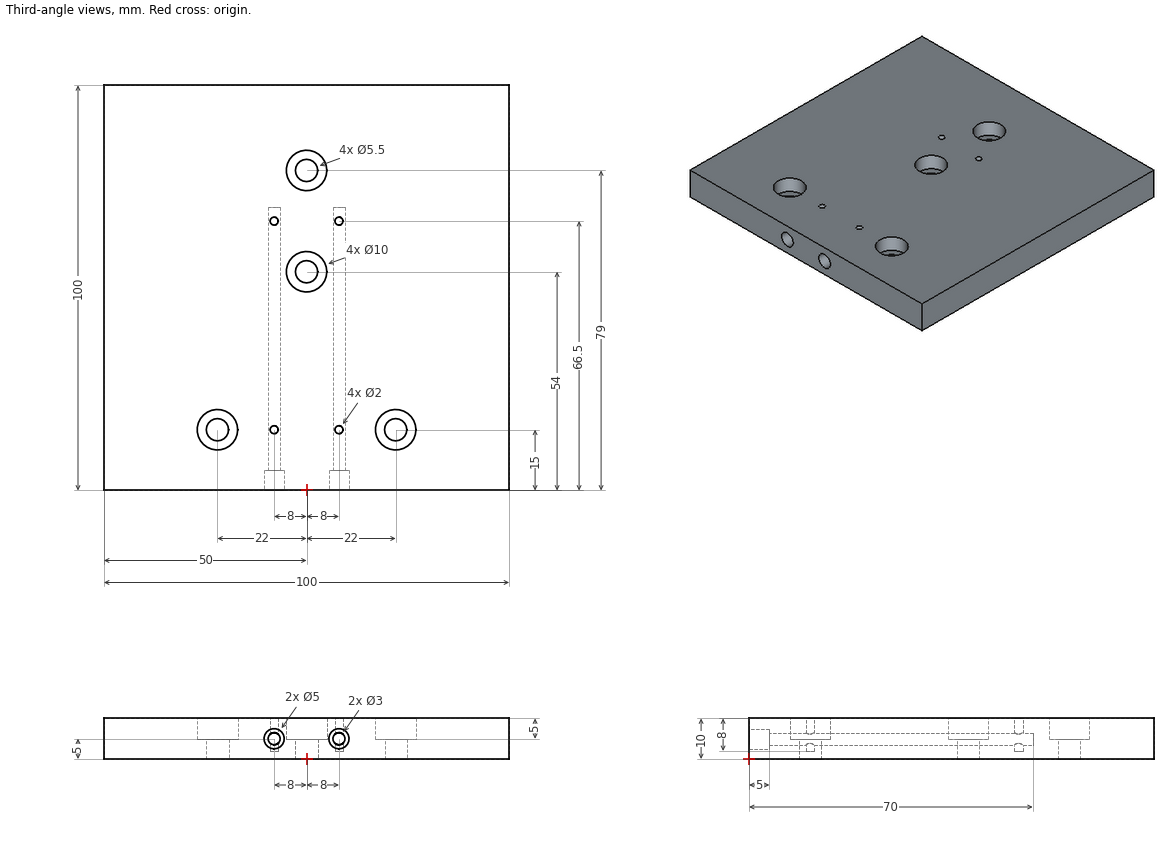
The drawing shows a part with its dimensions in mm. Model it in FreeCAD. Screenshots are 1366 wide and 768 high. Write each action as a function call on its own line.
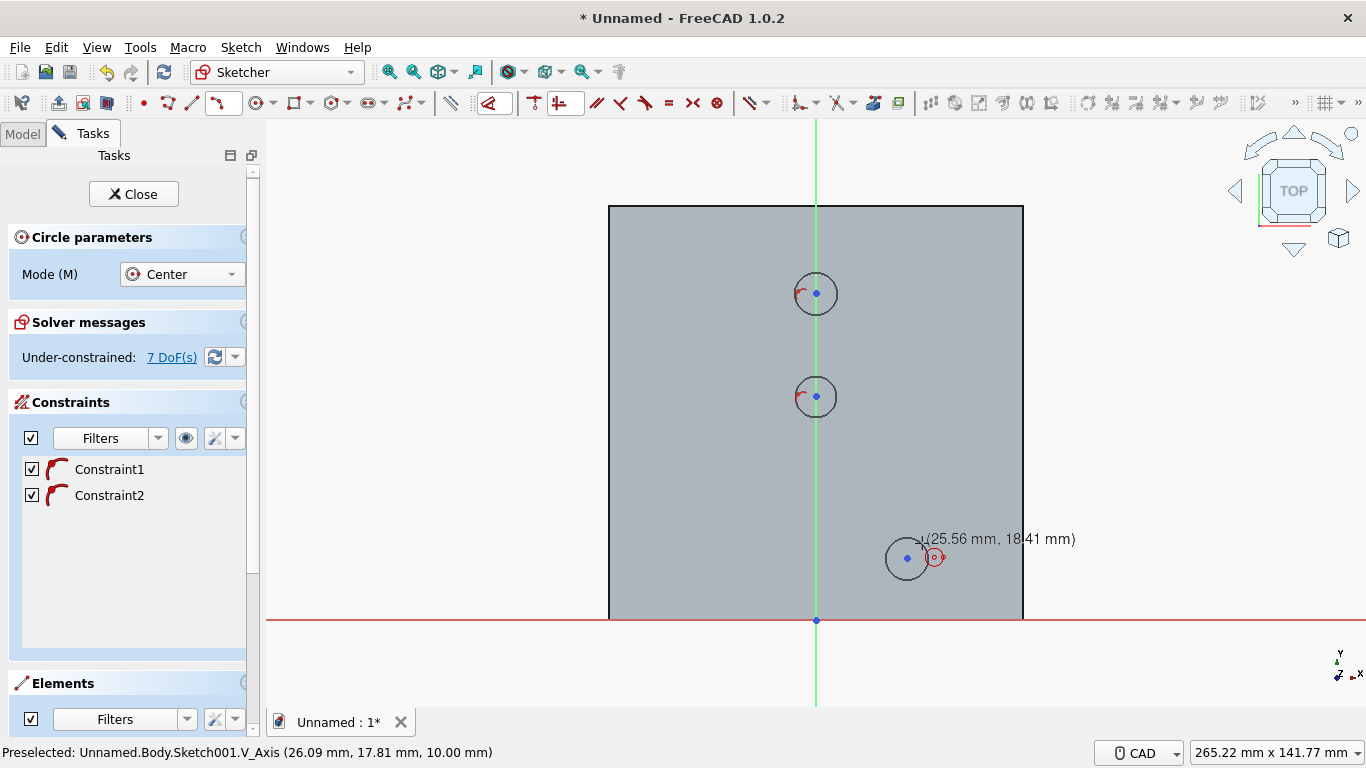
click(725, 558)
click(739, 543)
key(Escape)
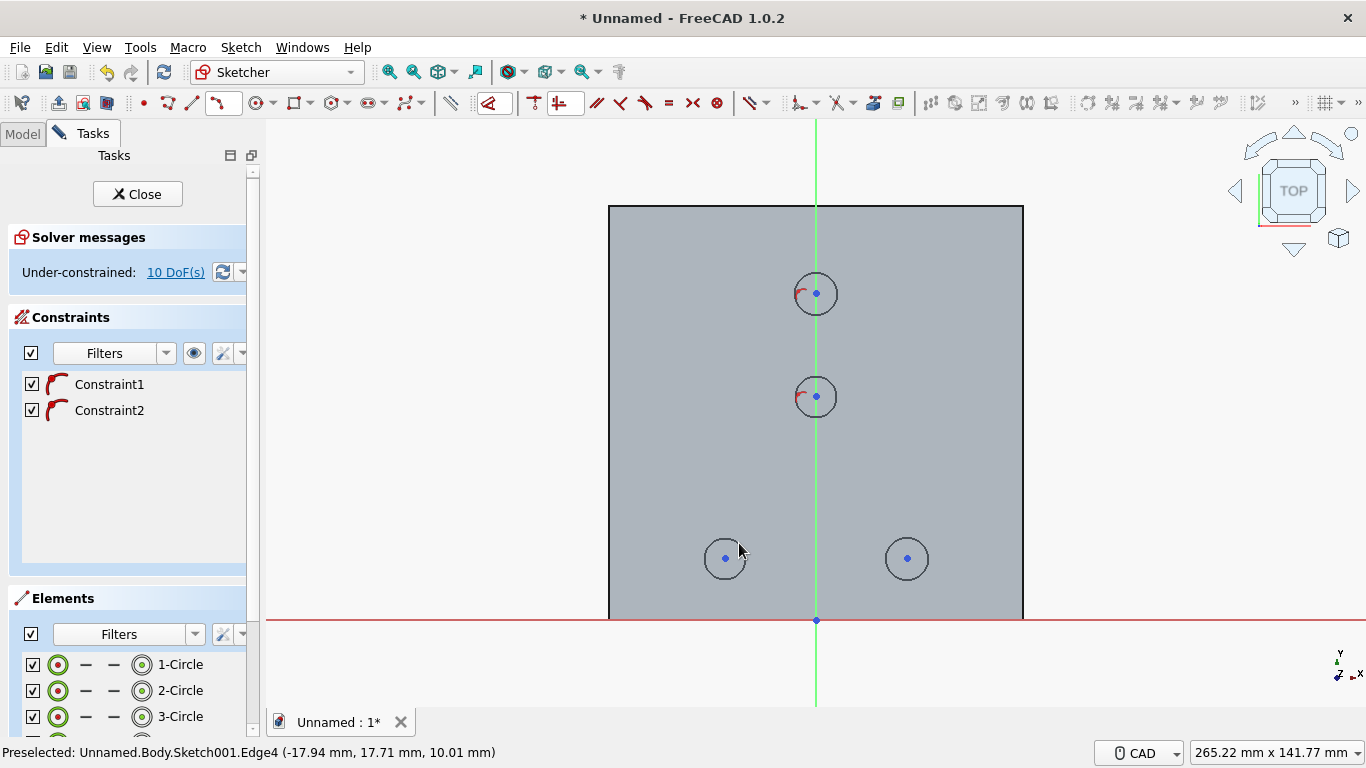
click(830, 382)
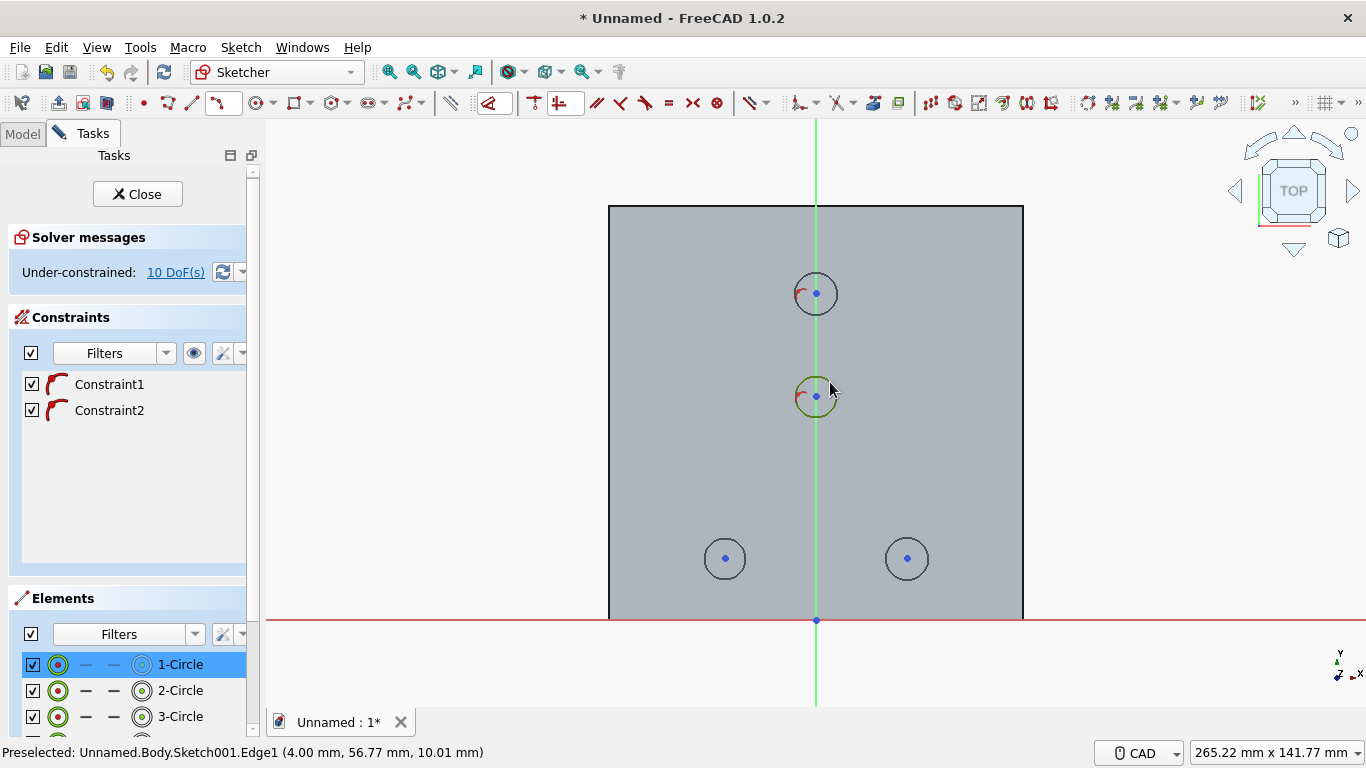
click(831, 279)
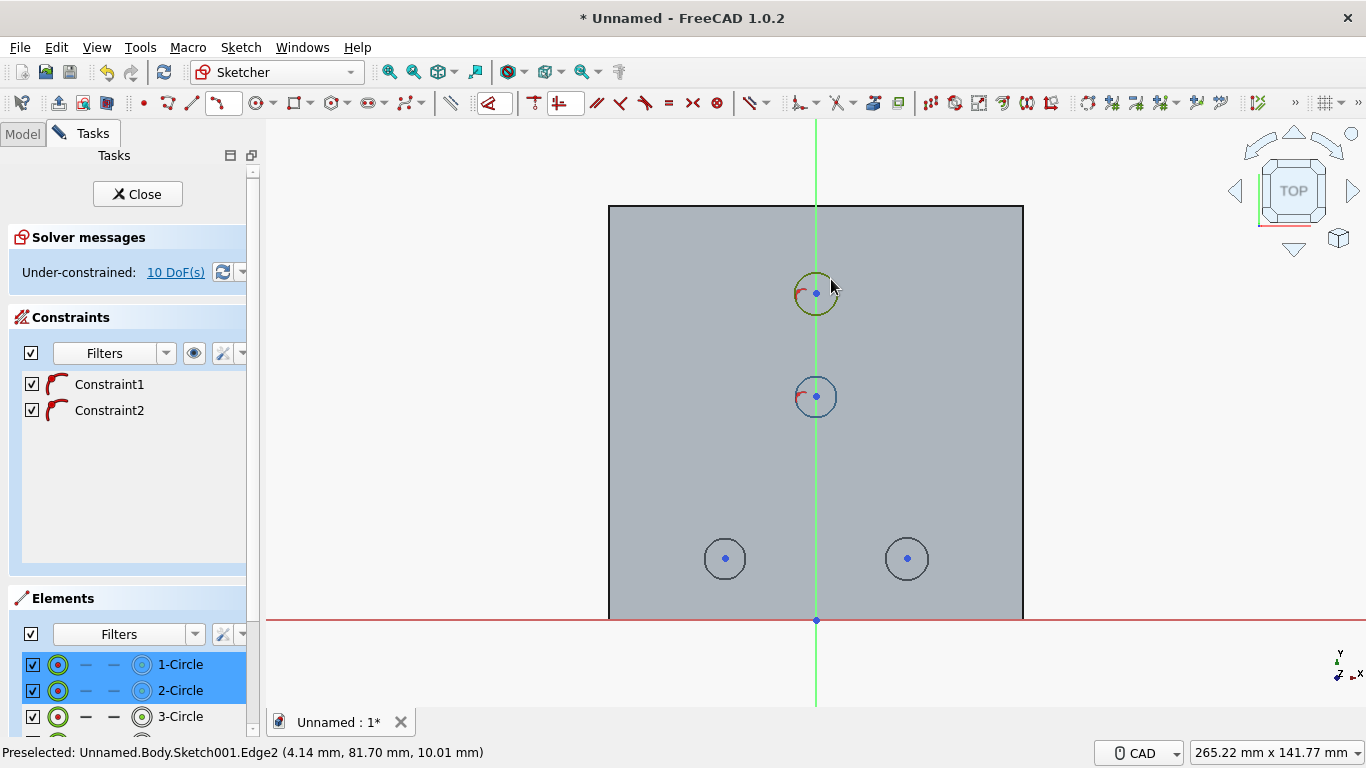
click(922, 544)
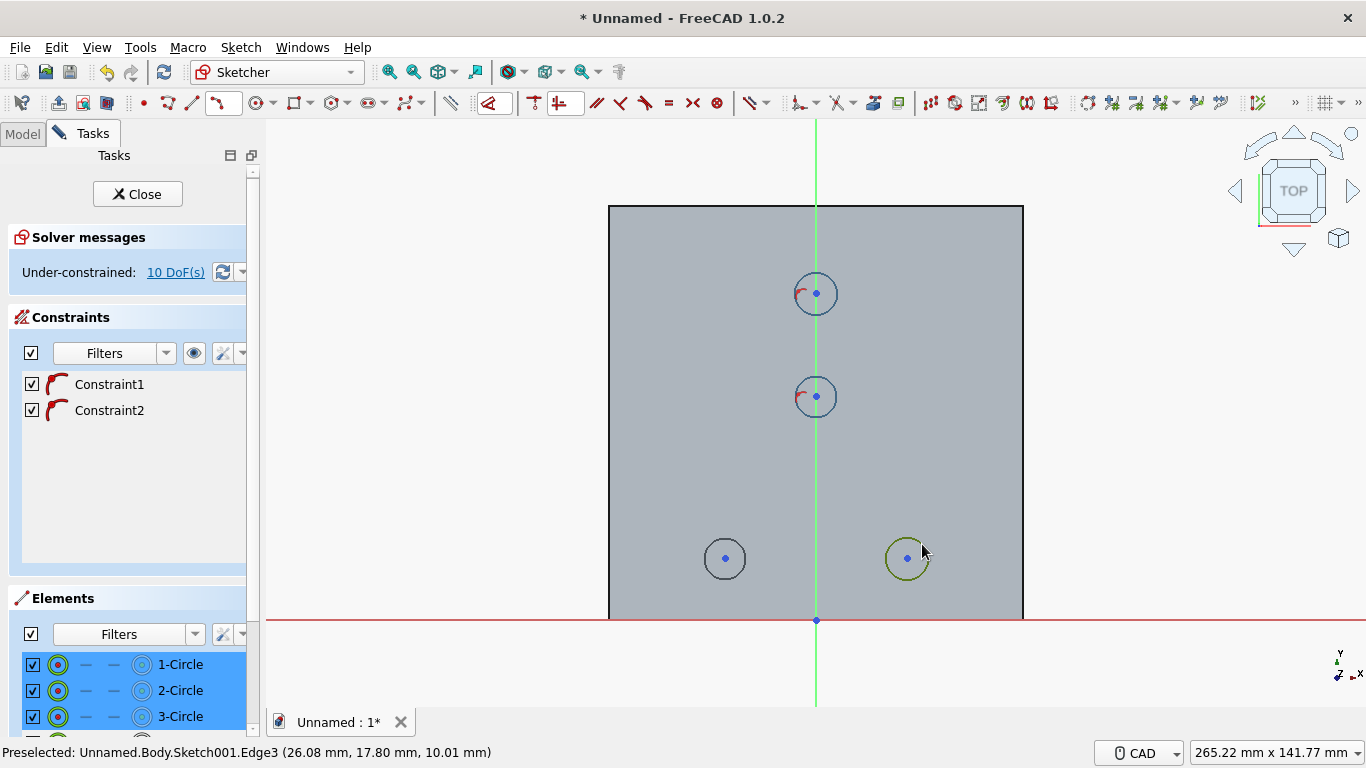
click(739, 544)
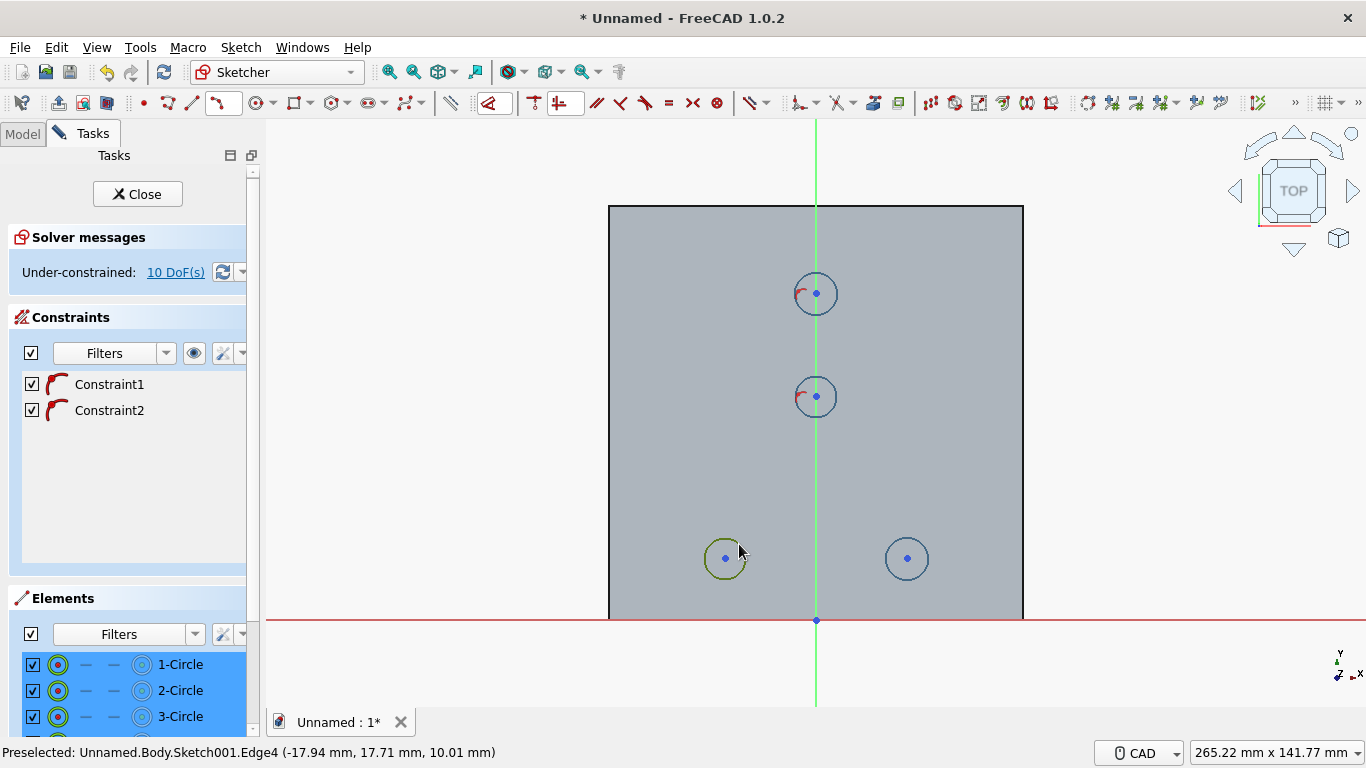
click(670, 104)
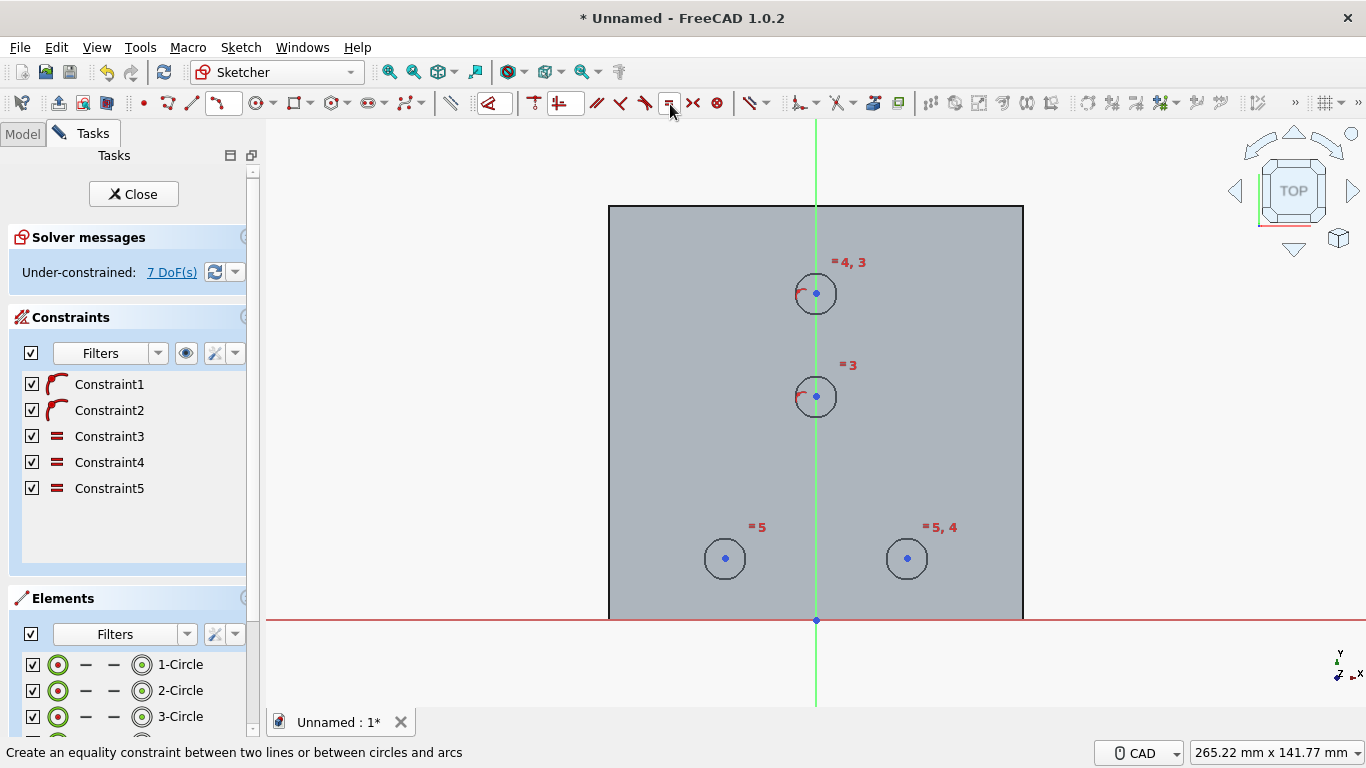
click(830, 382)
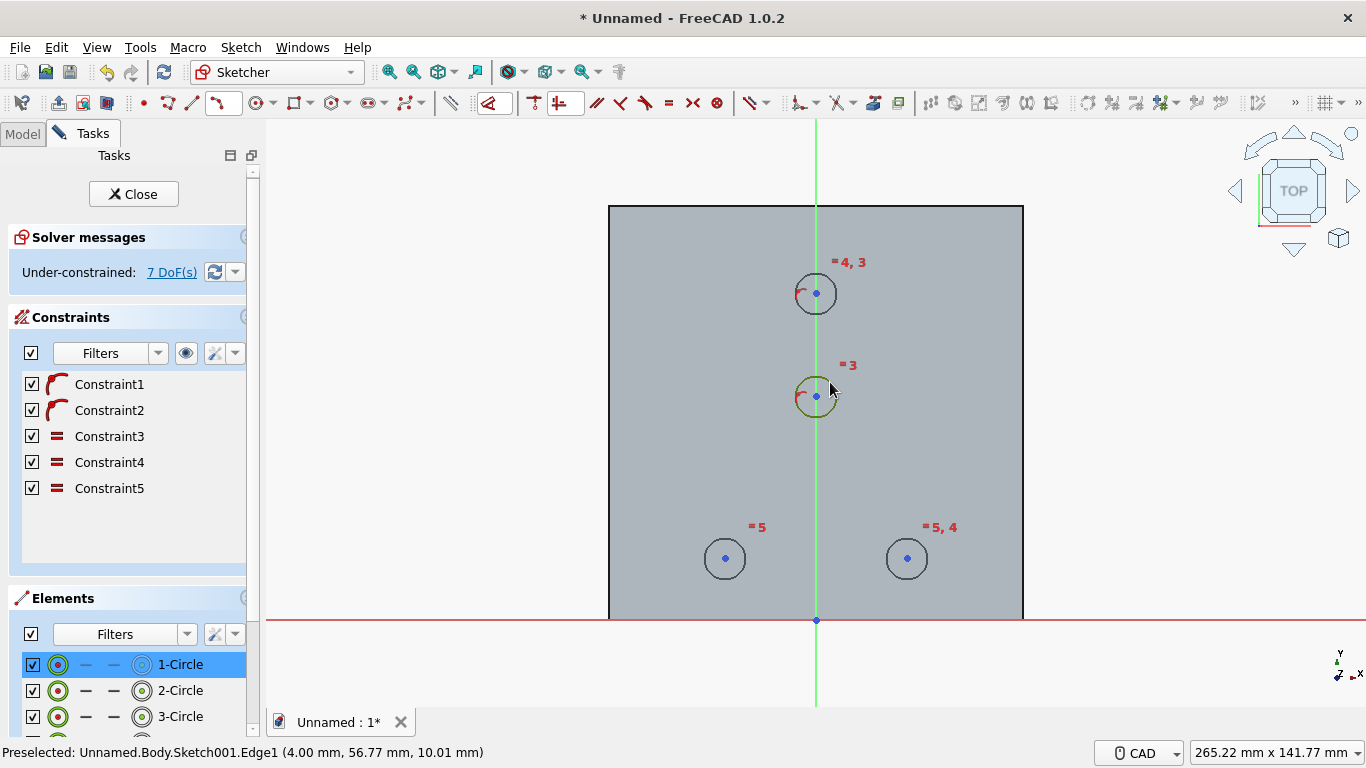
click(506, 104)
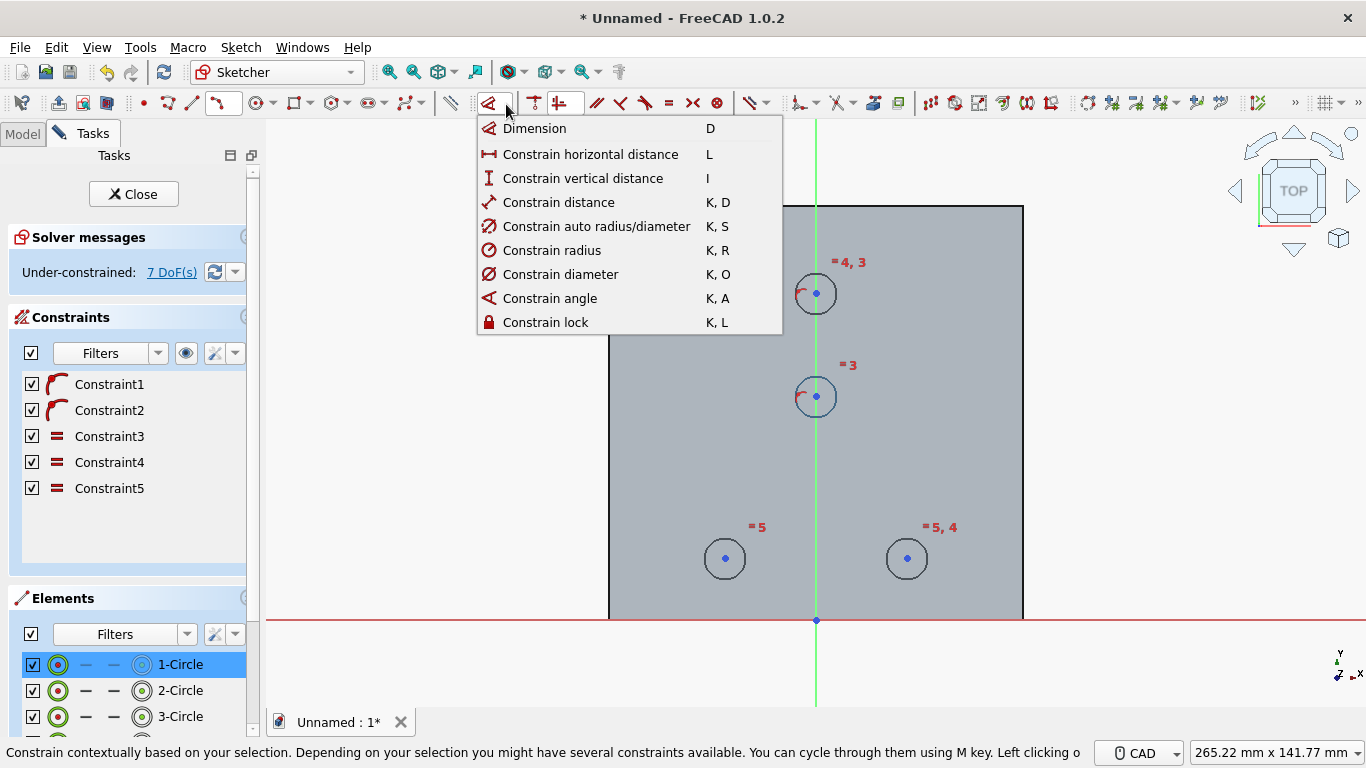
click(630, 274)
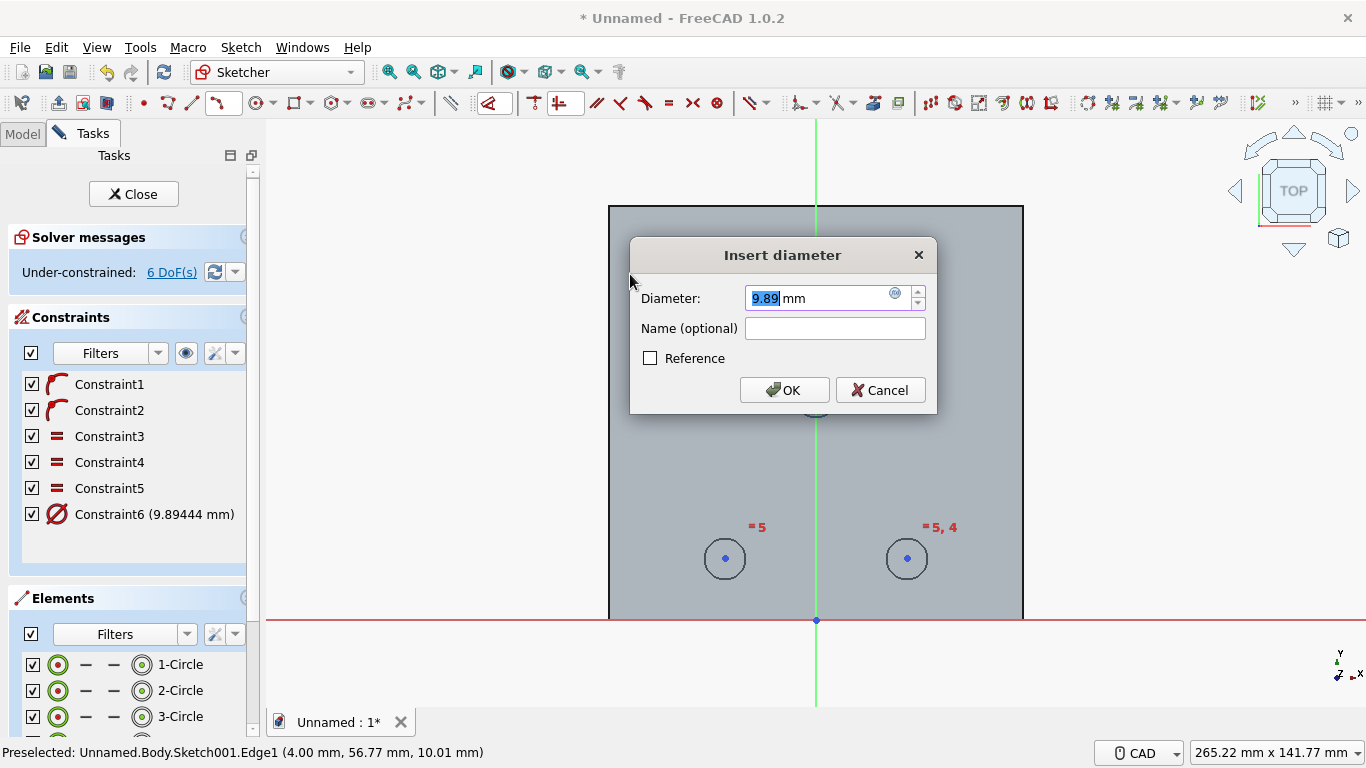
text(10)
key(Return)